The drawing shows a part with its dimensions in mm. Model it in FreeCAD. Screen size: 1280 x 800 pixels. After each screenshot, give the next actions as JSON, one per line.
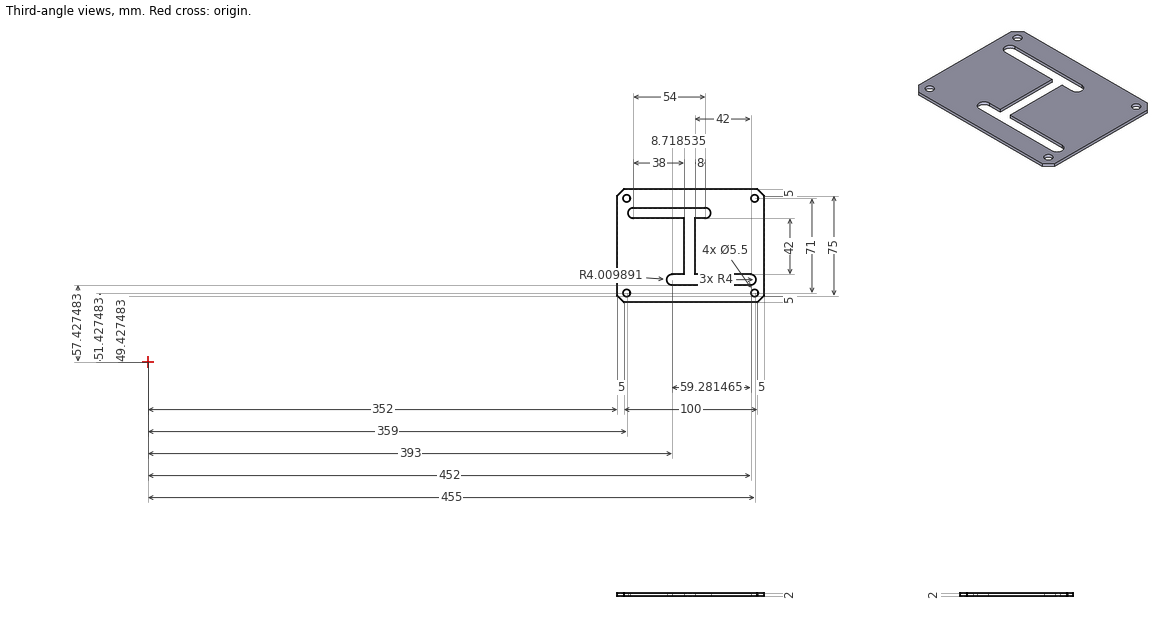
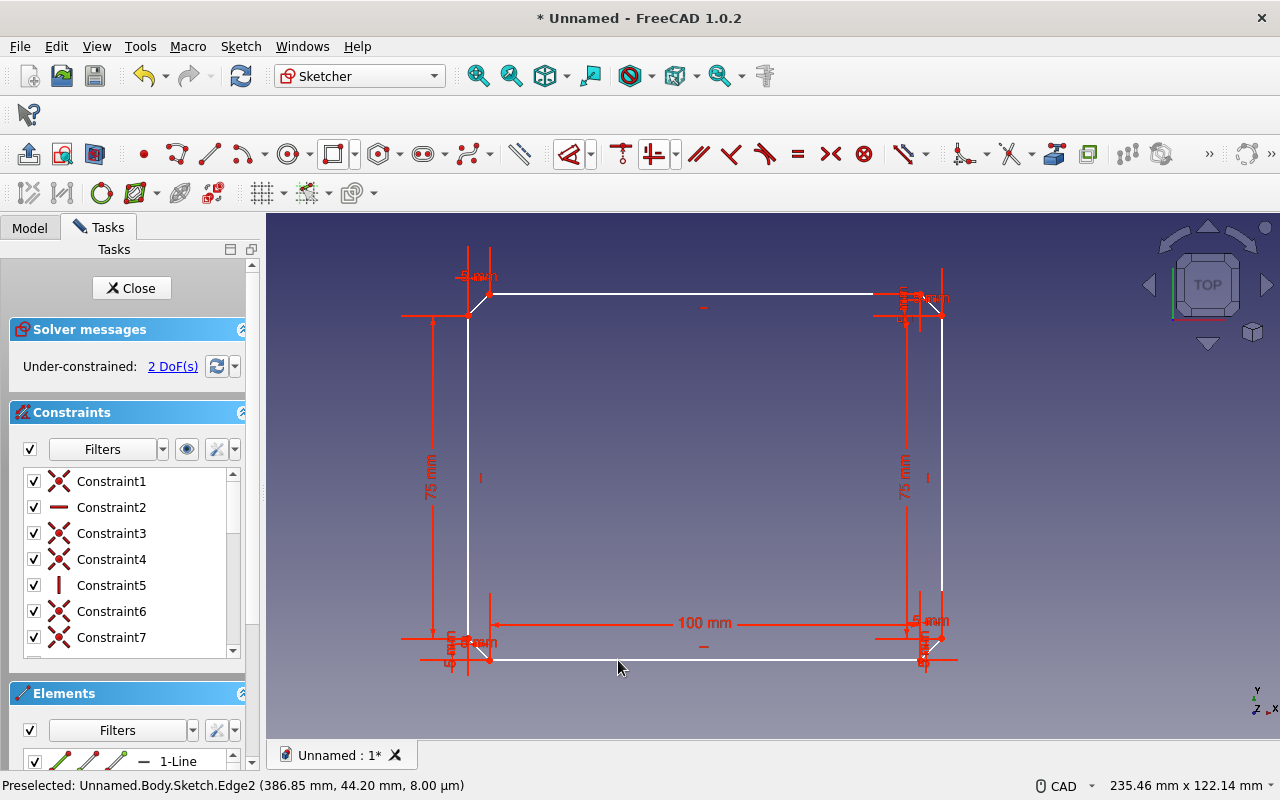
{"action": "left_click", "coordinate": [468, 639]}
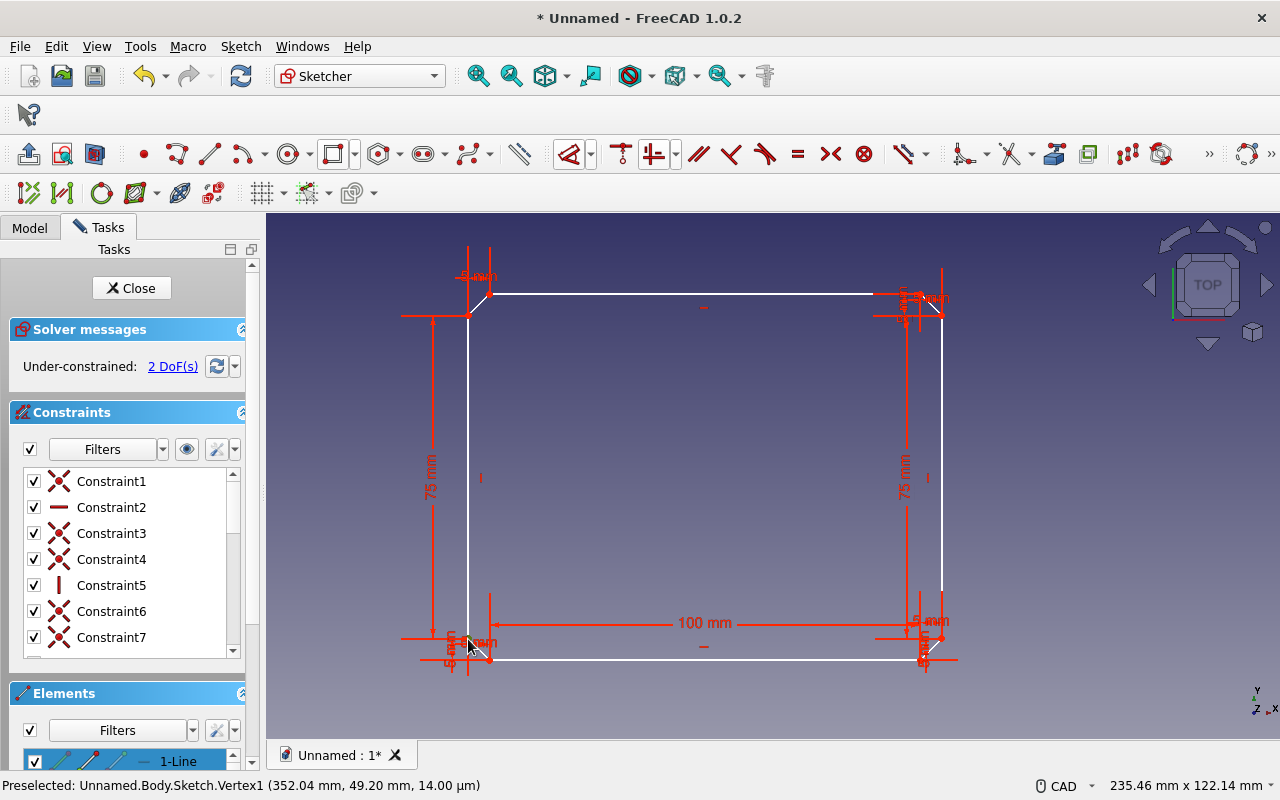
{"action": "key", "text": "l"}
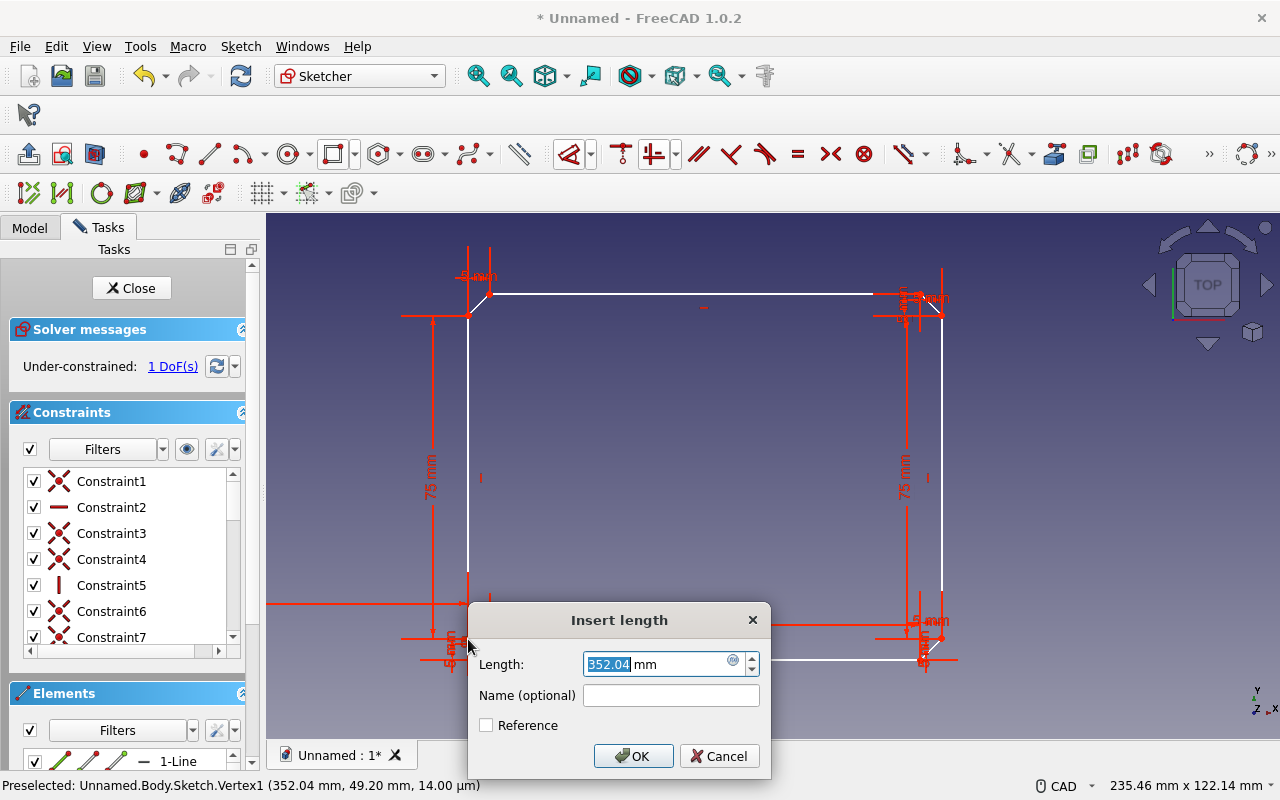
{"action": "type", "text": "352"}
{"action": "key", "text": "Return"}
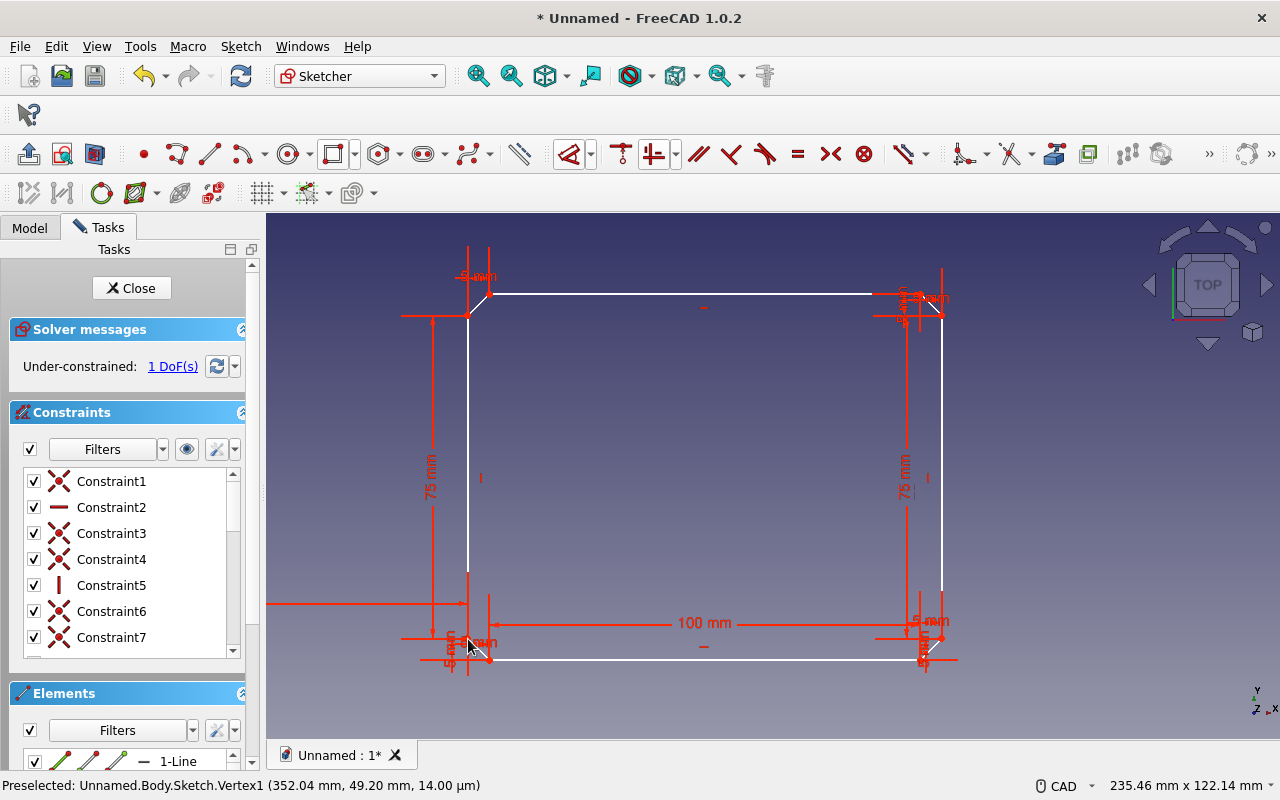
{"action": "left_click", "coordinate": [468, 639]}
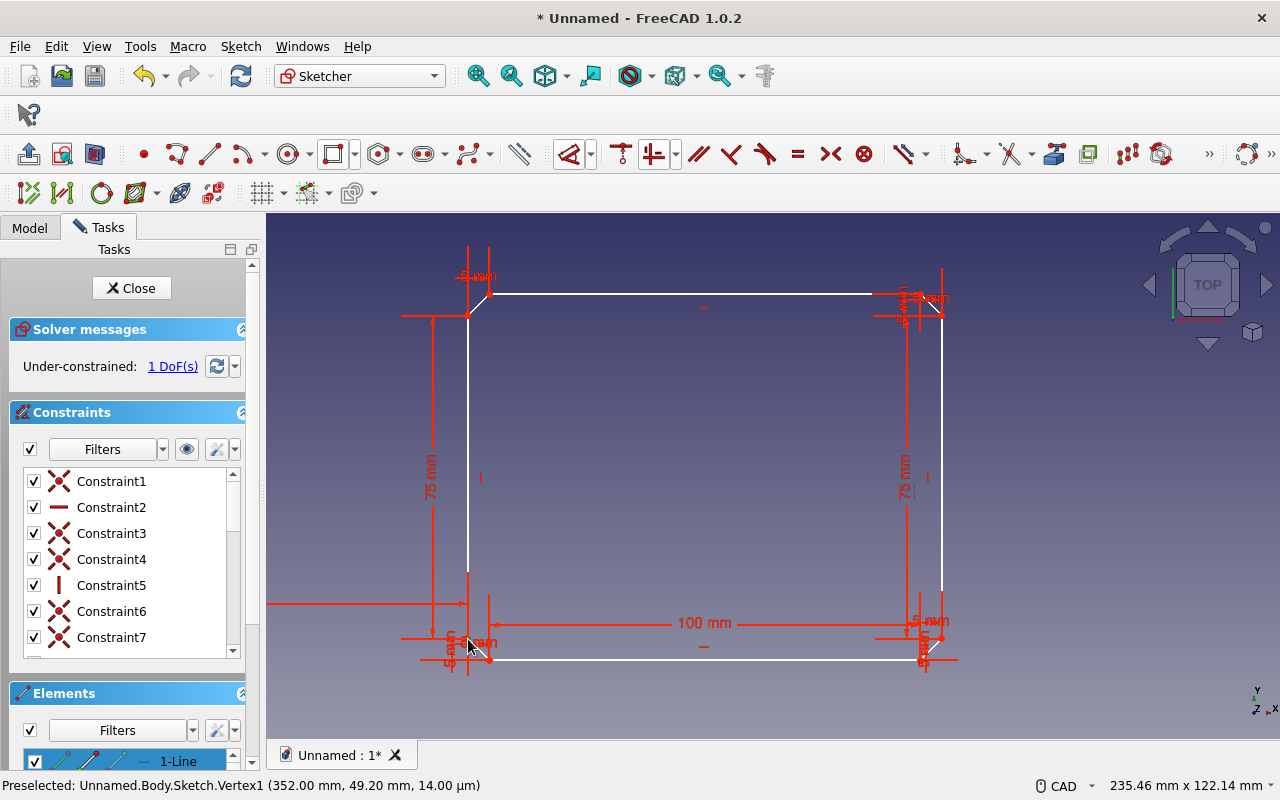
{"action": "key", "text": "i"}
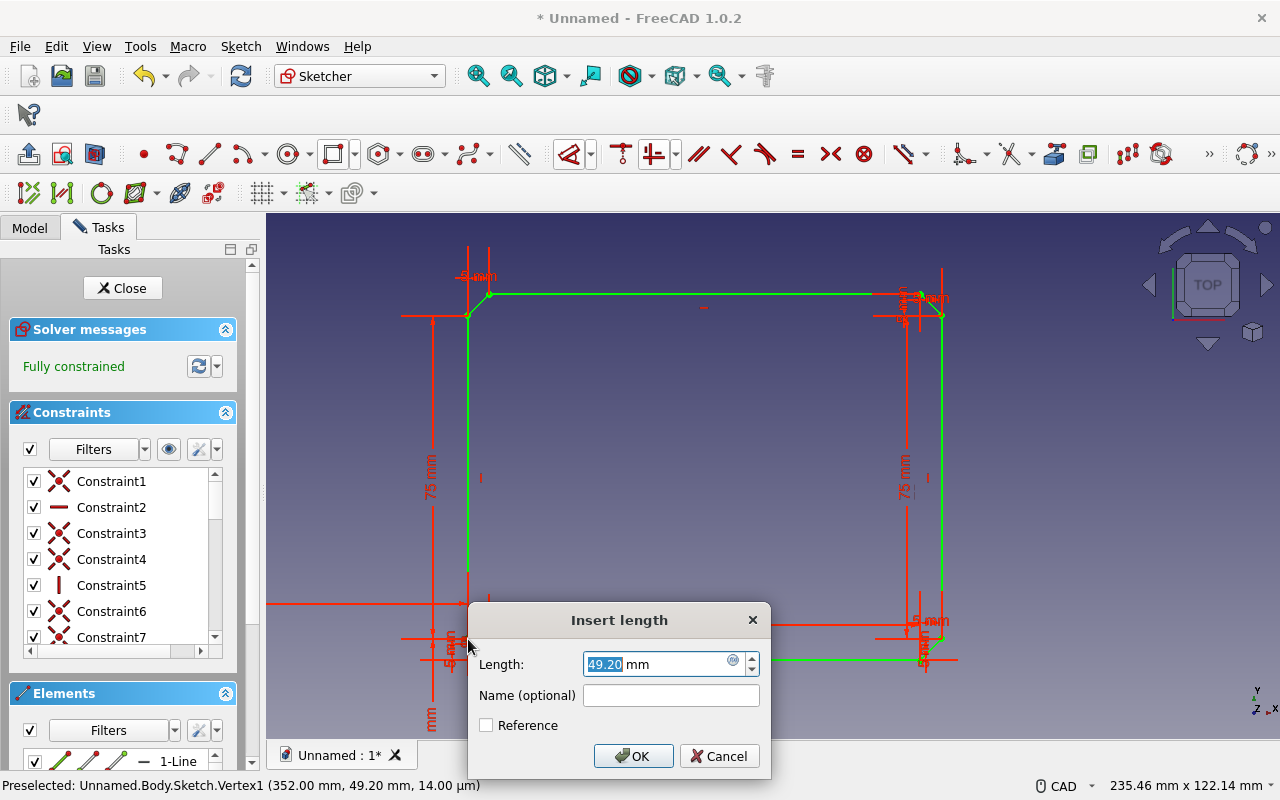
{"action": "type", "text": "49.427483"}
{"action": "key", "text": "Return"}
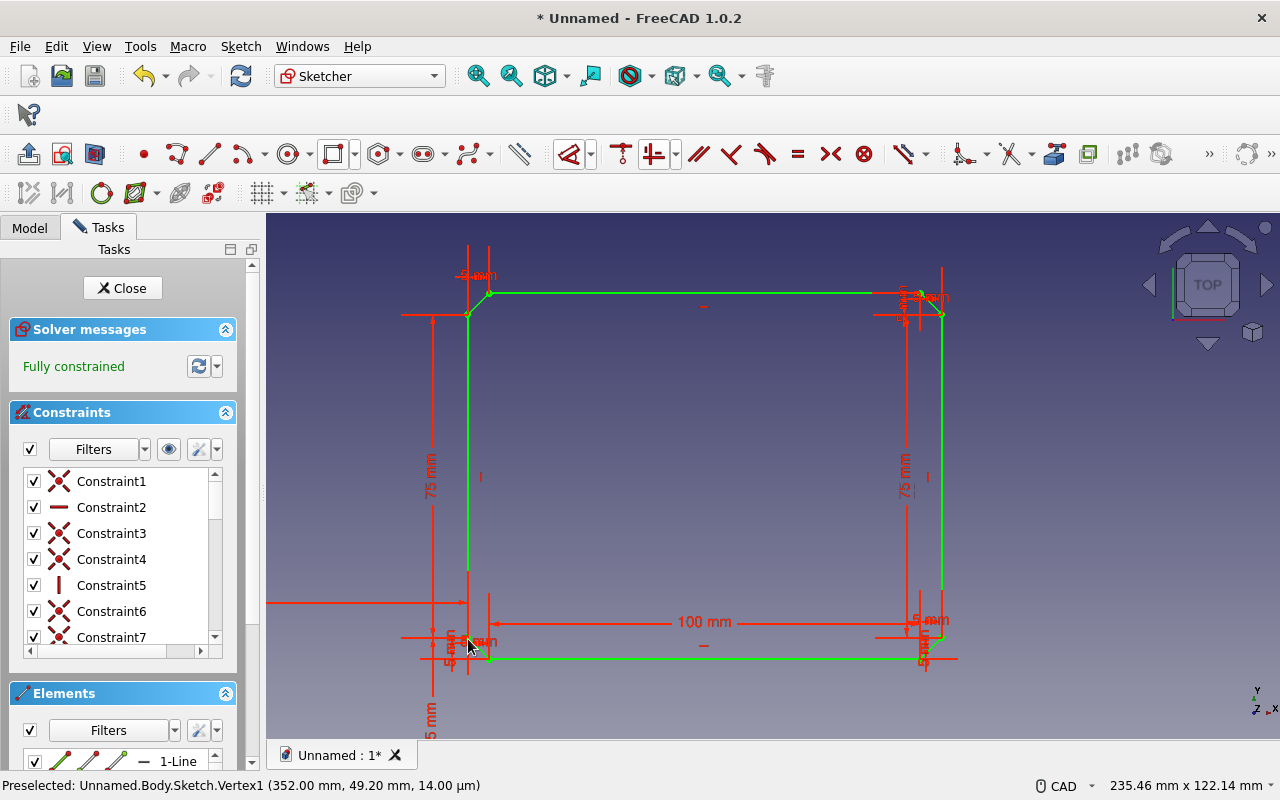
{"action": "left_click", "coordinate": [123, 288]}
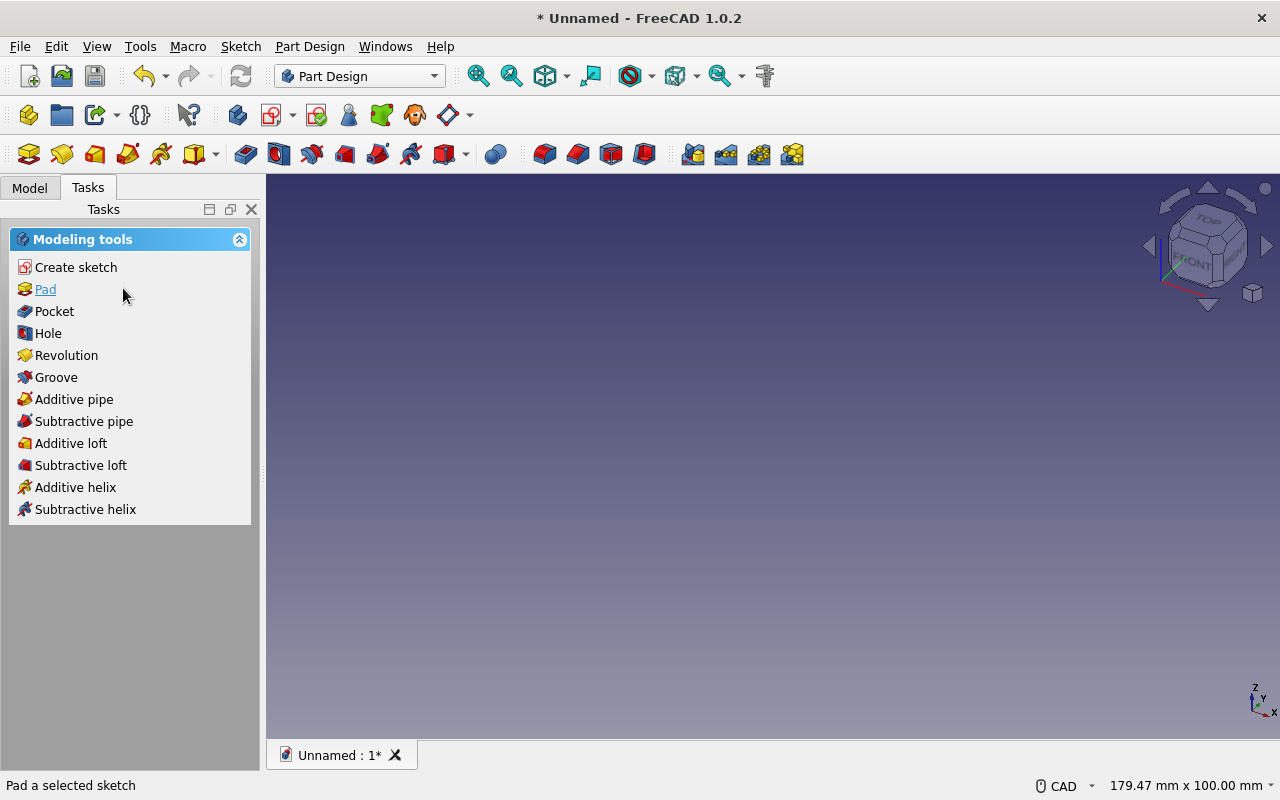
{"action": "left_click", "coordinate": [29, 154]}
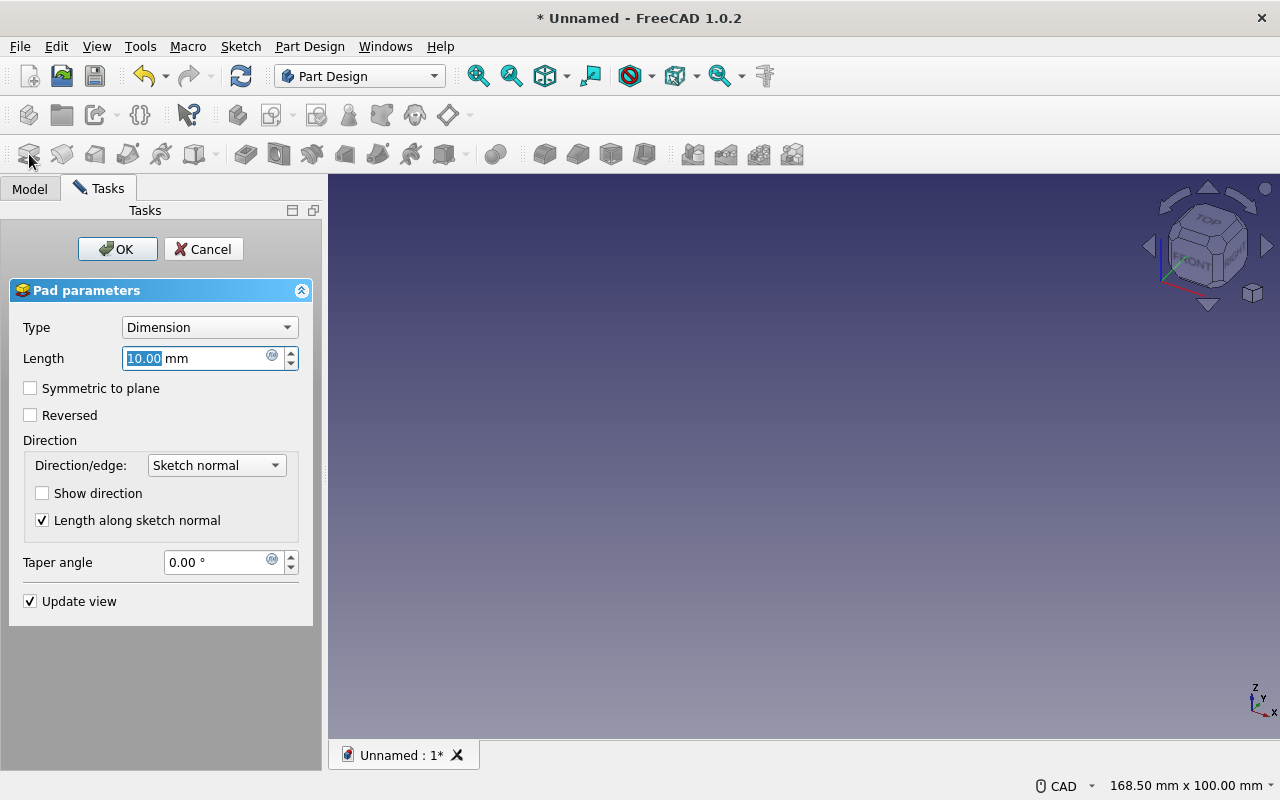
{"action": "type", "text": "2"}
{"action": "key", "text": "Tab"}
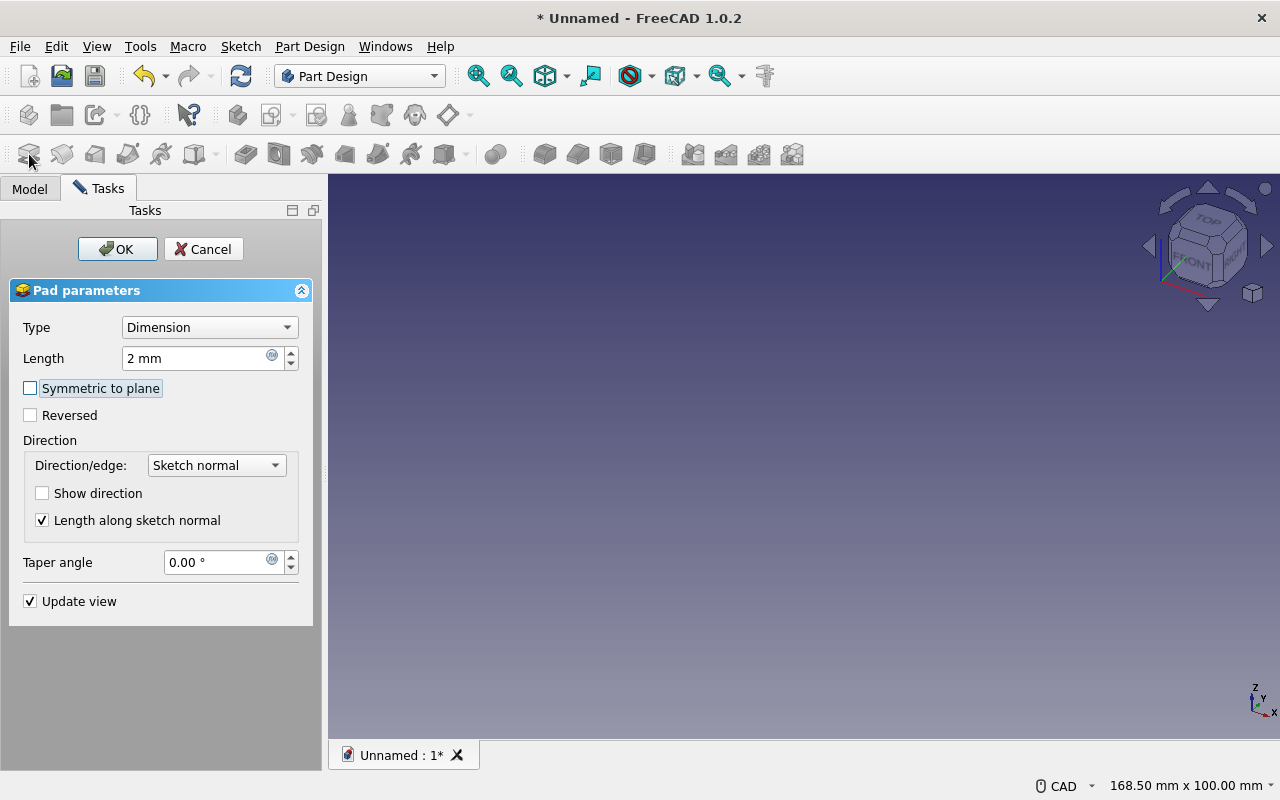
{"action": "left_click", "coordinate": [118, 249]}